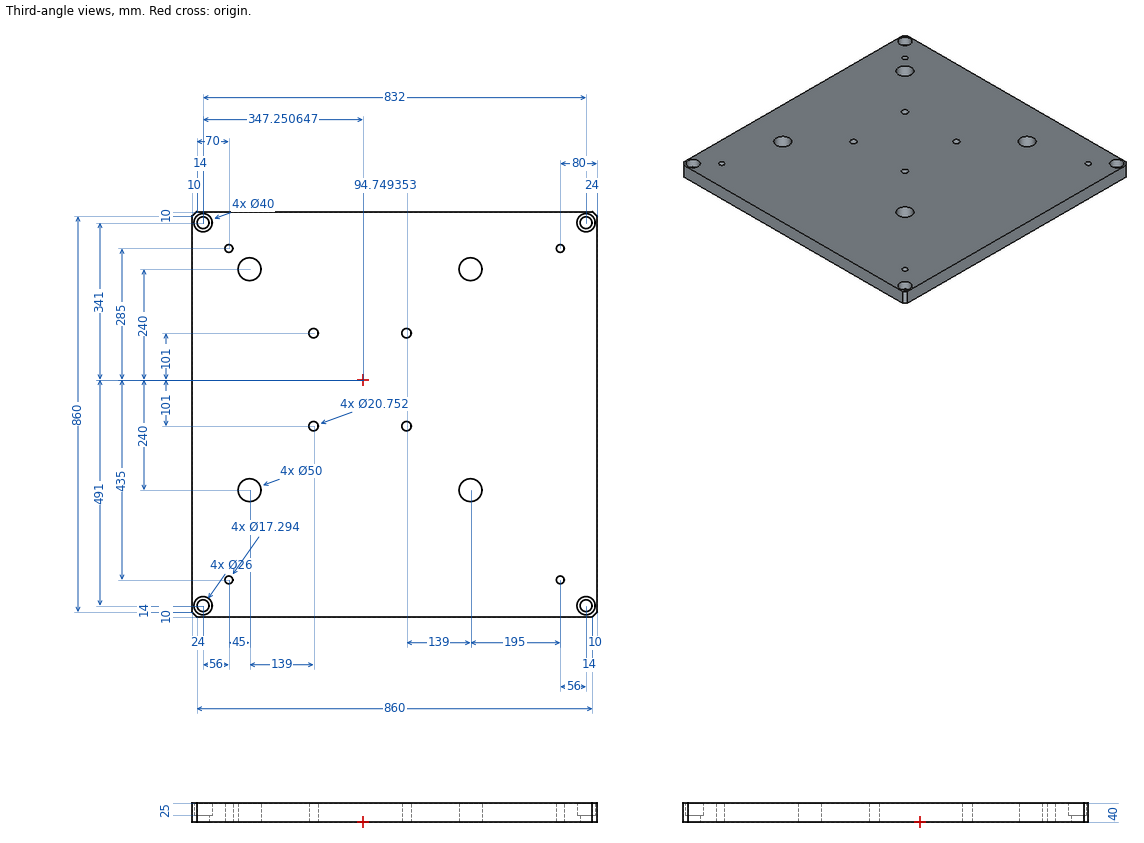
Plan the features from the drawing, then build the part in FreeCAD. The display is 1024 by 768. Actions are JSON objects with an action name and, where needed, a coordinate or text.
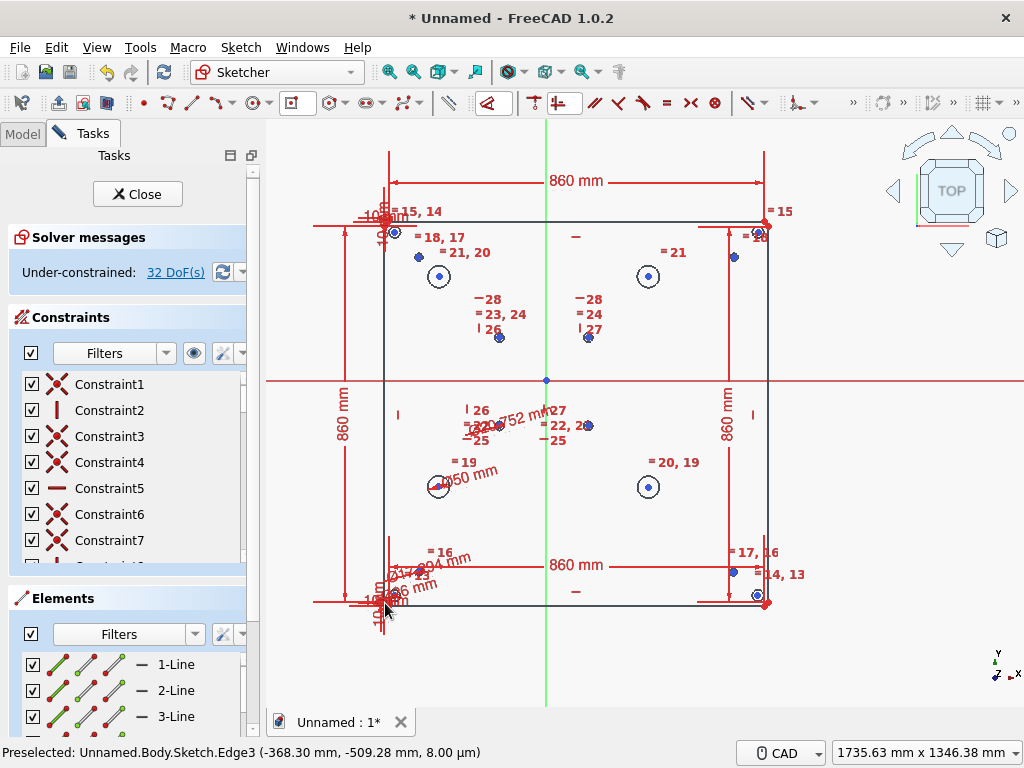
{"action": "scroll", "coordinate": [765, 605], "scroll_direction": "up", "scroll_amount": 12}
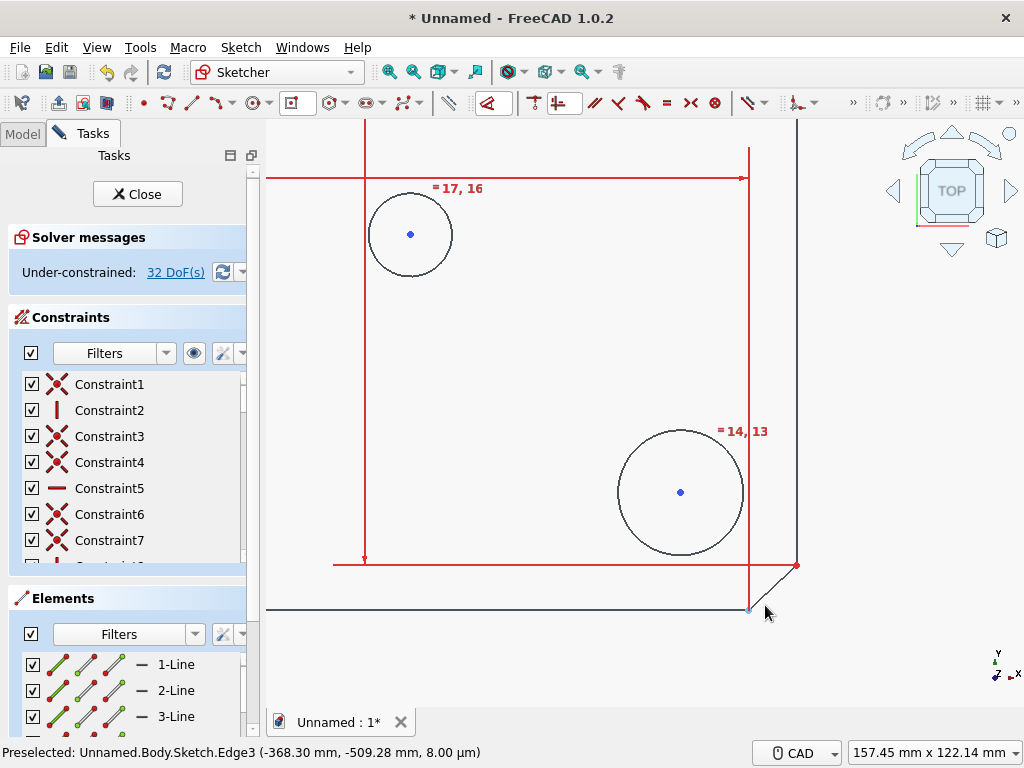
{"action": "left_click", "coordinate": [763, 597]}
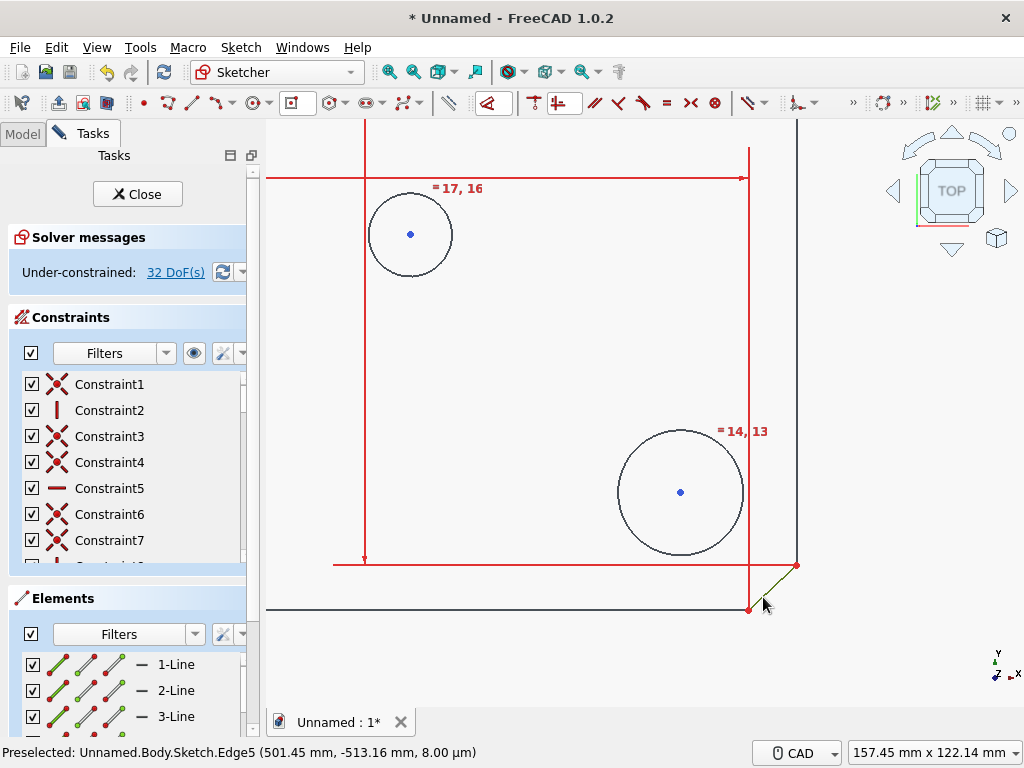
{"action": "key", "text": "l"}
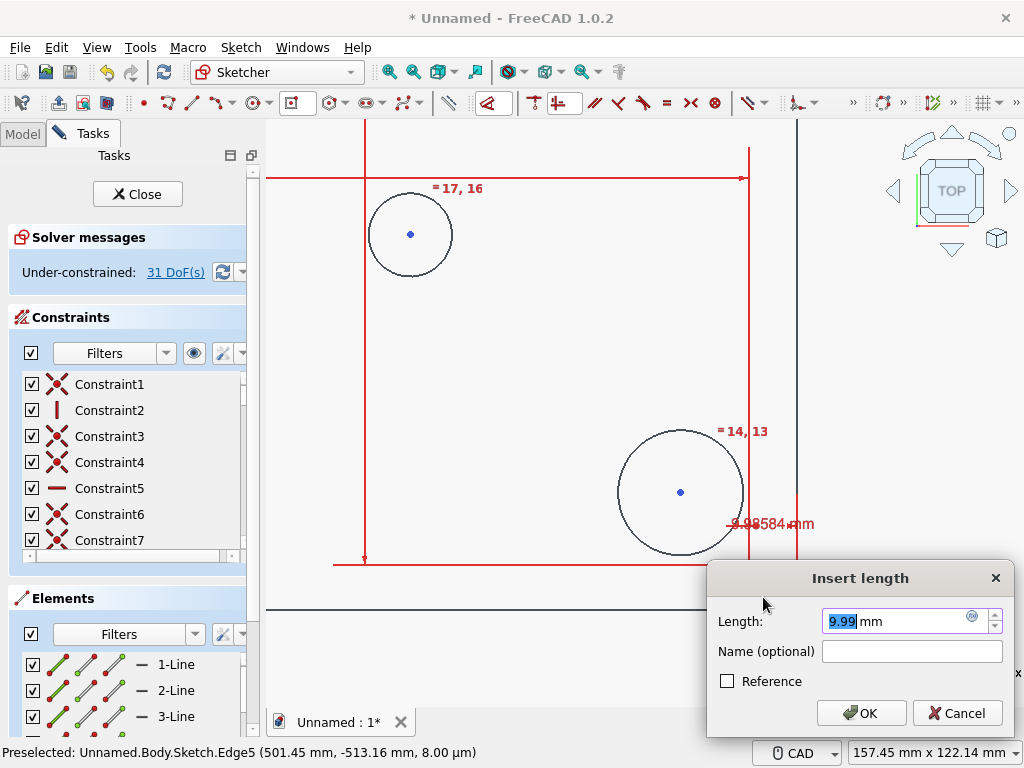
{"action": "type", "text": "10"}
{"action": "key", "text": "Return"}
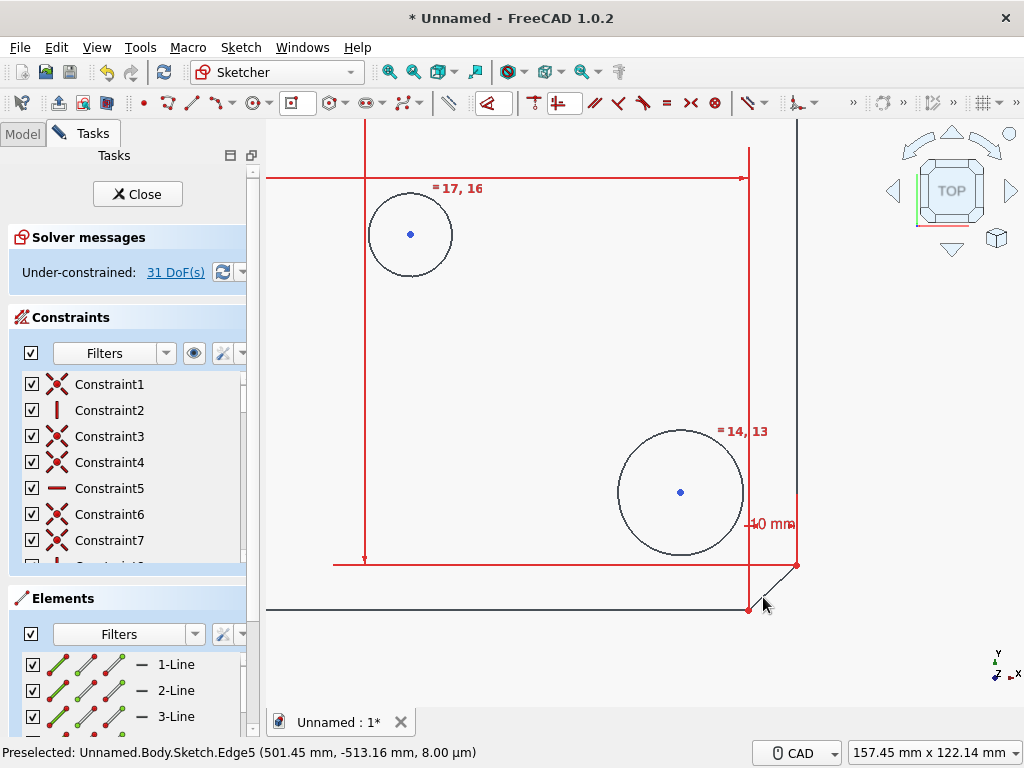
{"action": "left_click", "coordinate": [763, 597]}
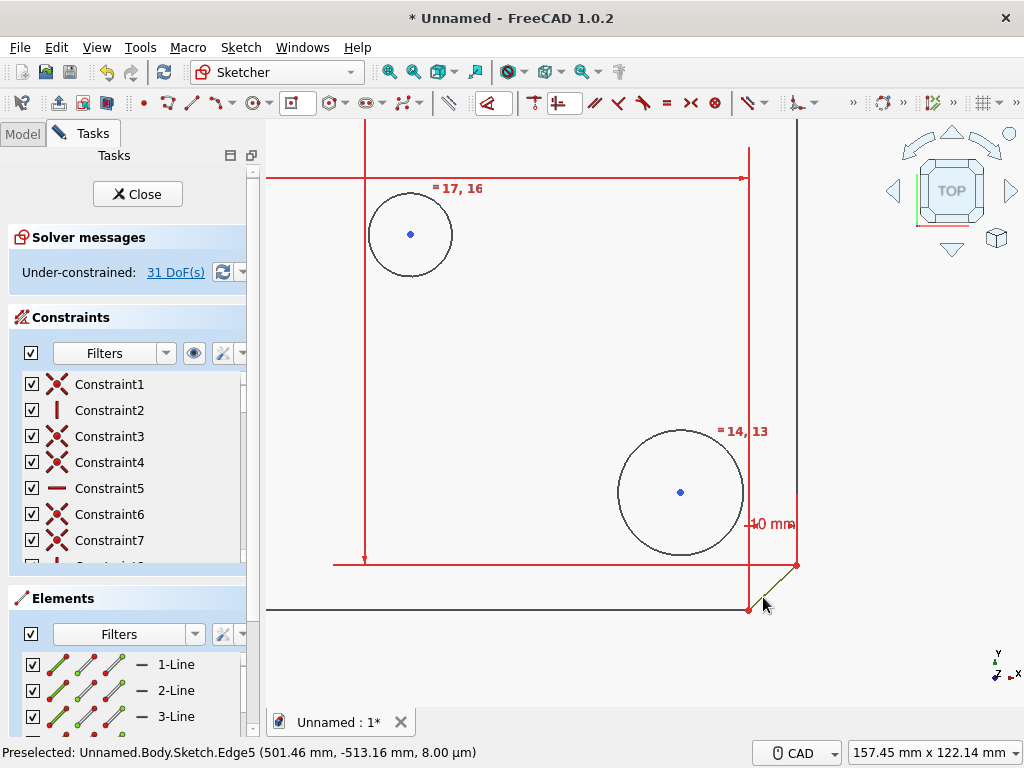
{"action": "left_click", "coordinate": [506, 104]}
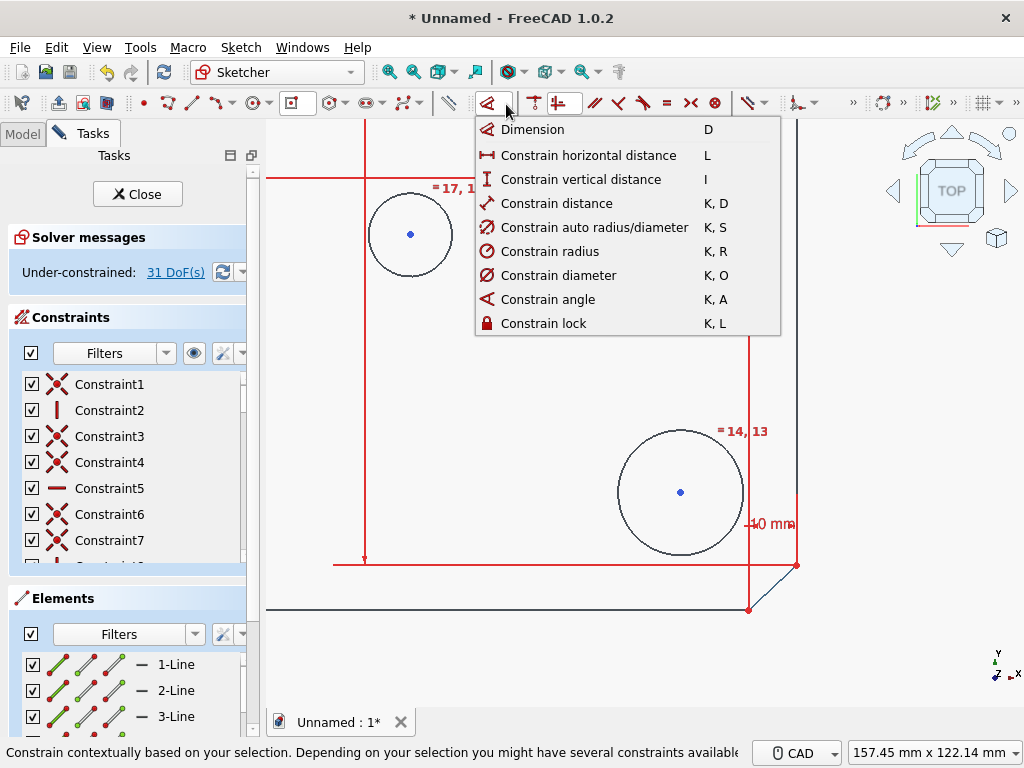
{"action": "left_click", "coordinate": [628, 179]}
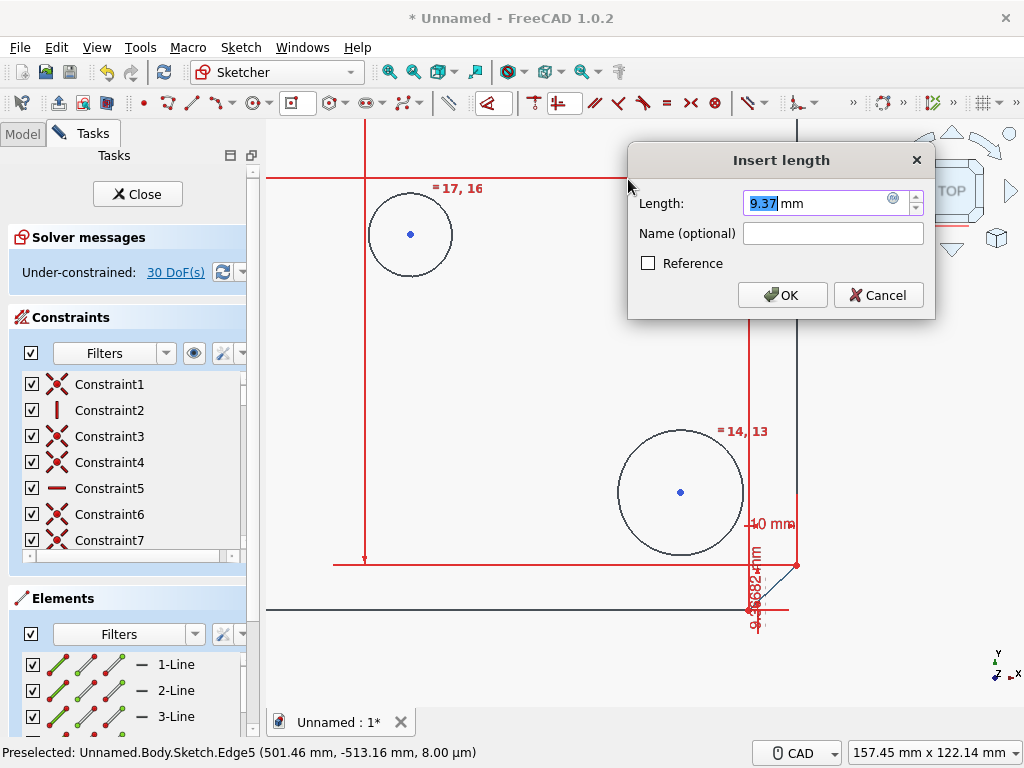
{"action": "type", "text": "10"}
{"action": "key", "text": "Return"}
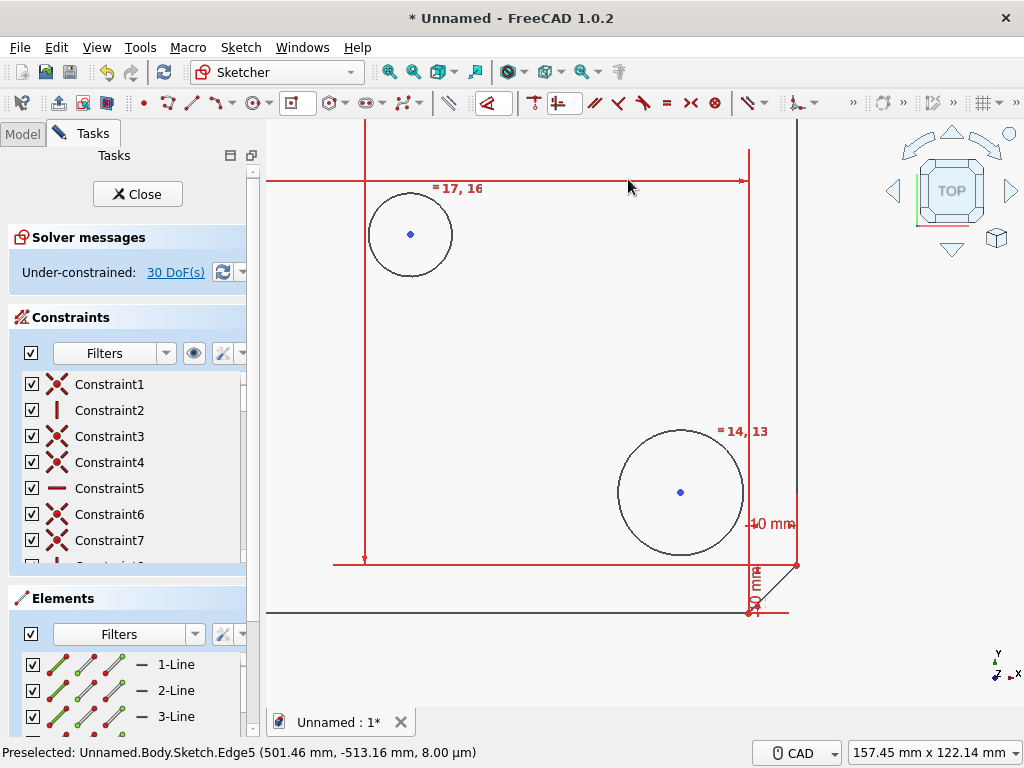
{"action": "scroll", "coordinate": [766, 605], "scroll_direction": "down", "scroll_amount": 12}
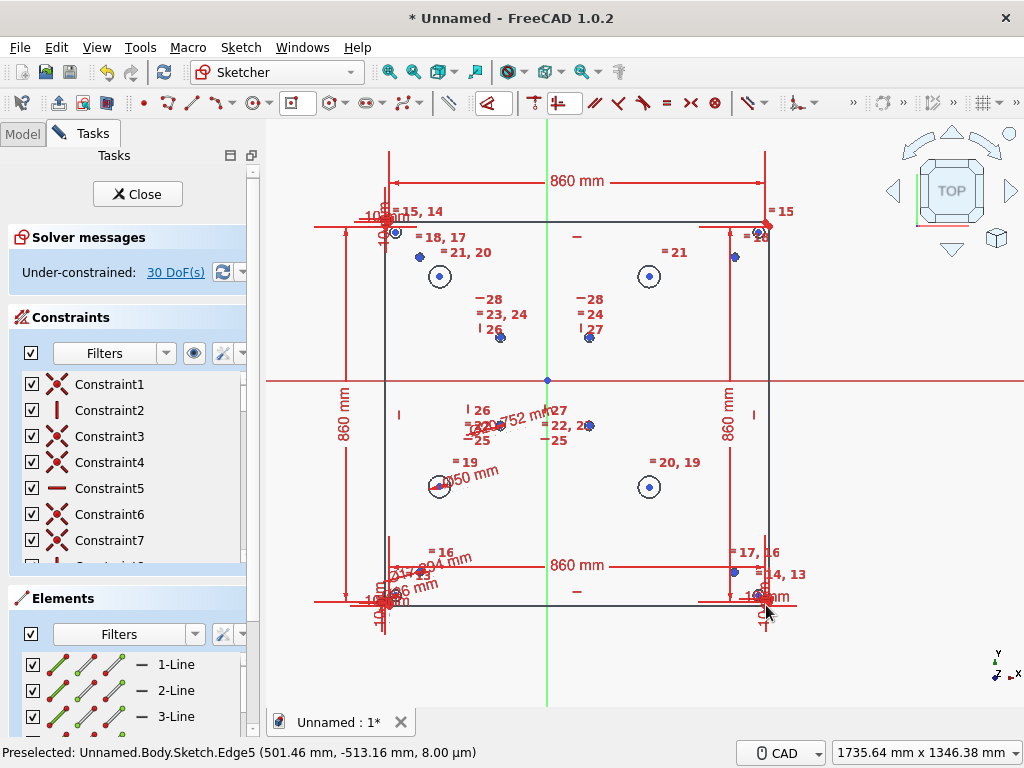
{"action": "left_click", "coordinate": [396, 596]}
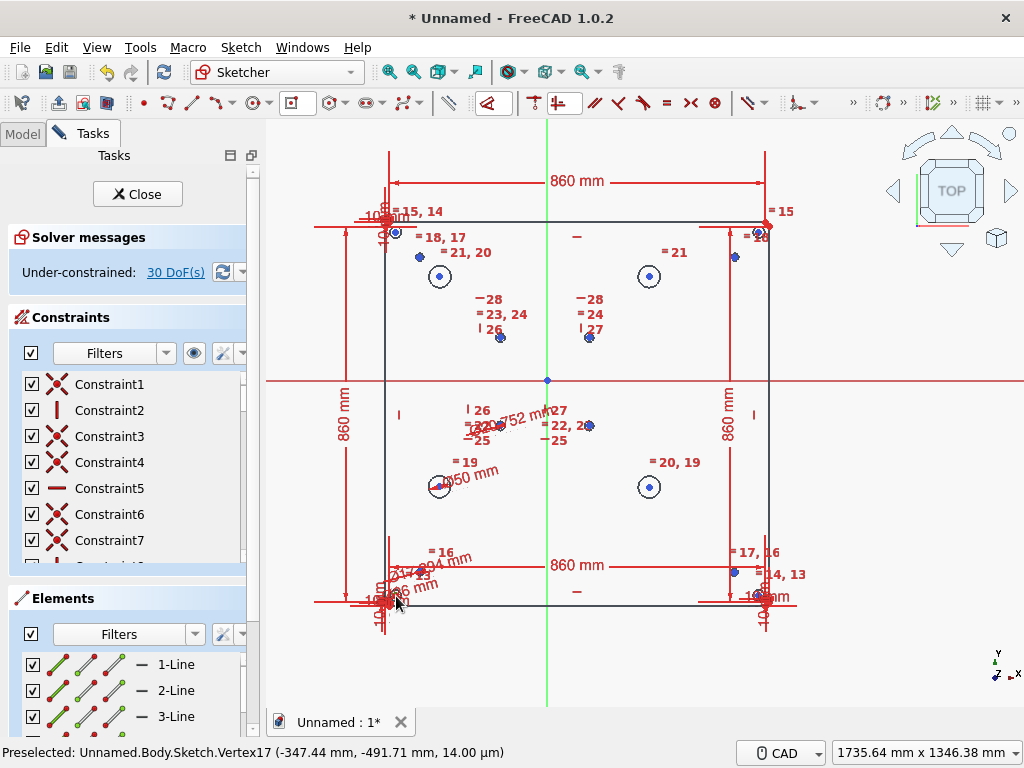
{"action": "key", "text": "i"}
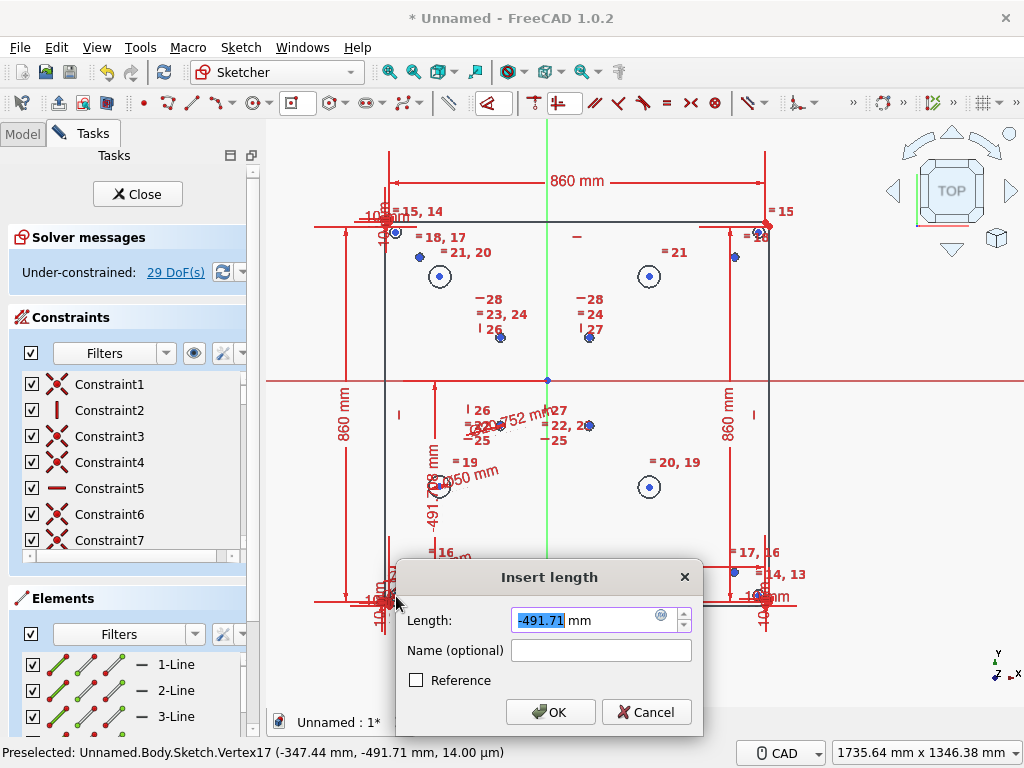
{"action": "type", "text": "-491"}
{"action": "key", "text": "Return"}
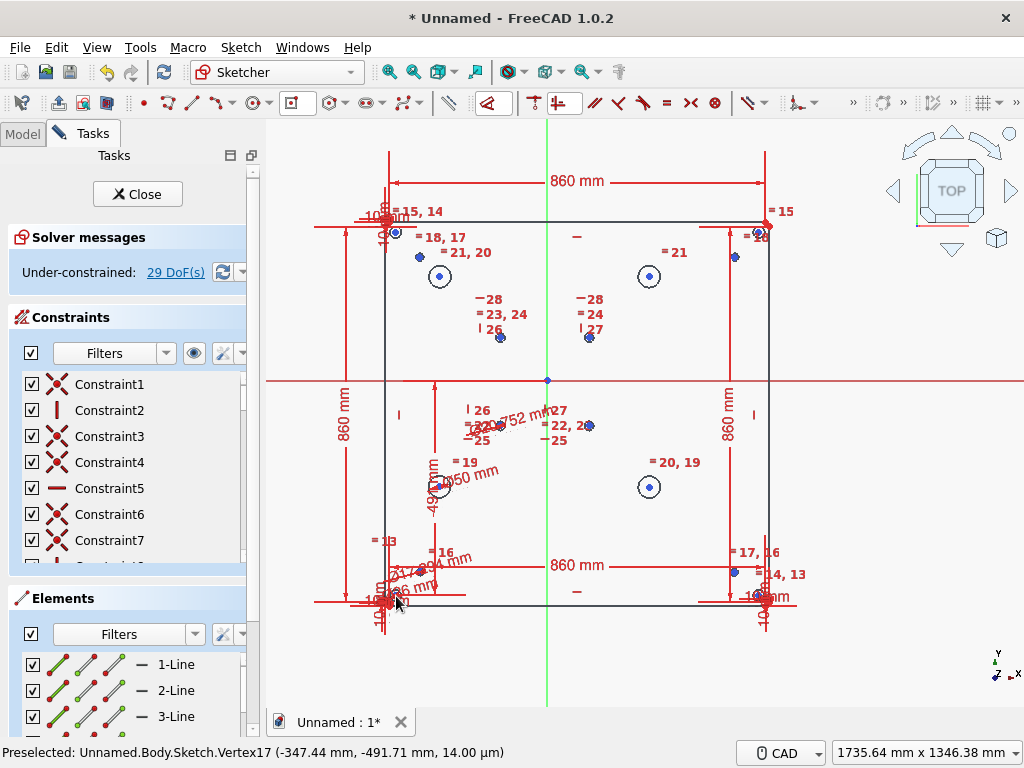
{"action": "left_click", "coordinate": [421, 572]}